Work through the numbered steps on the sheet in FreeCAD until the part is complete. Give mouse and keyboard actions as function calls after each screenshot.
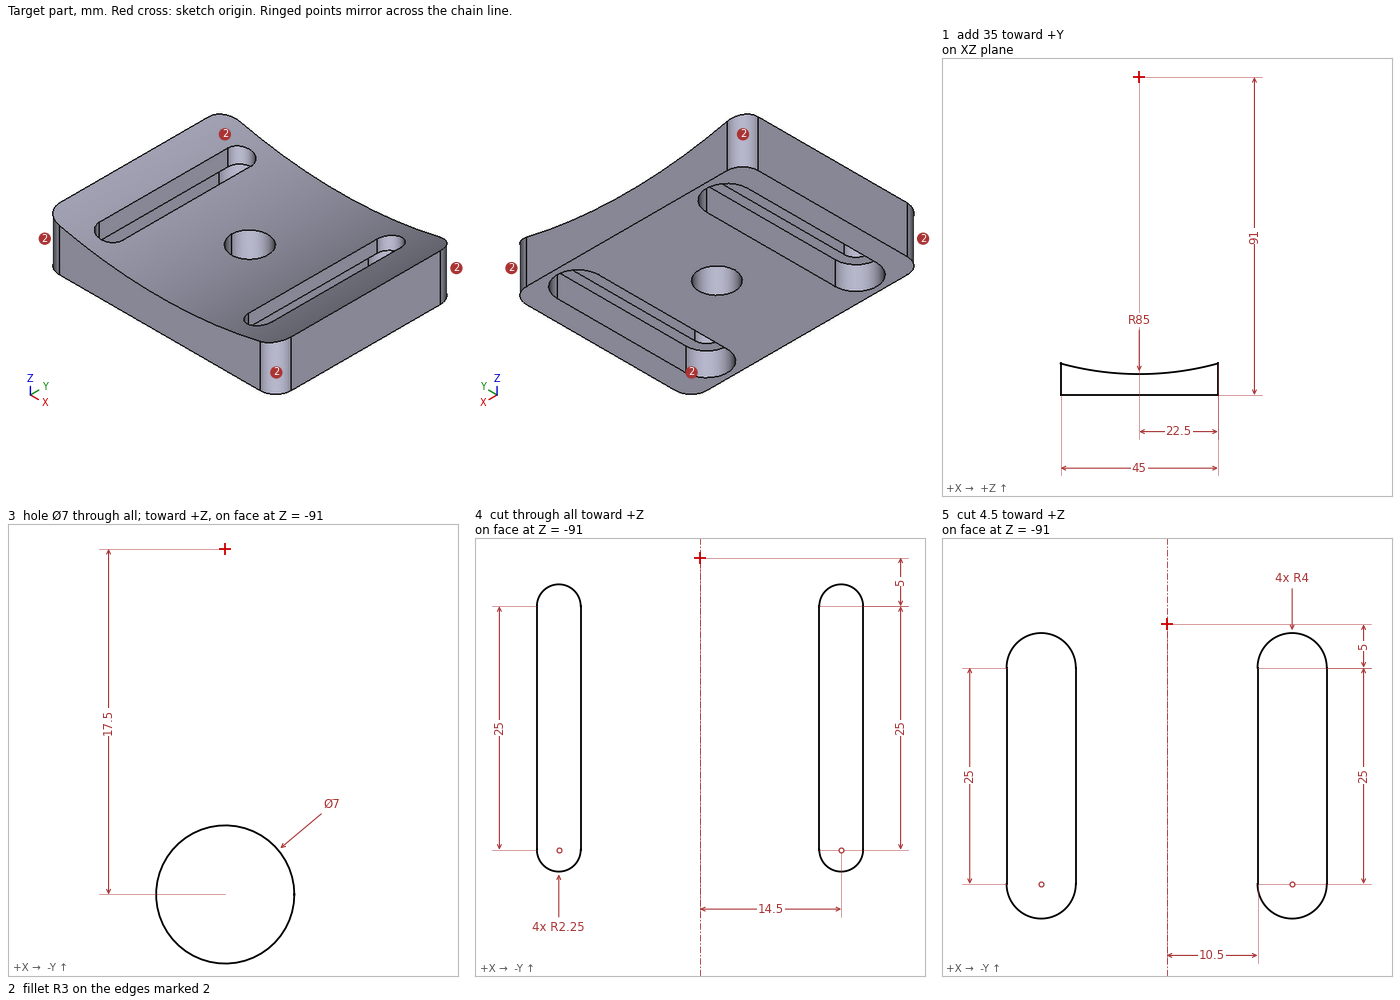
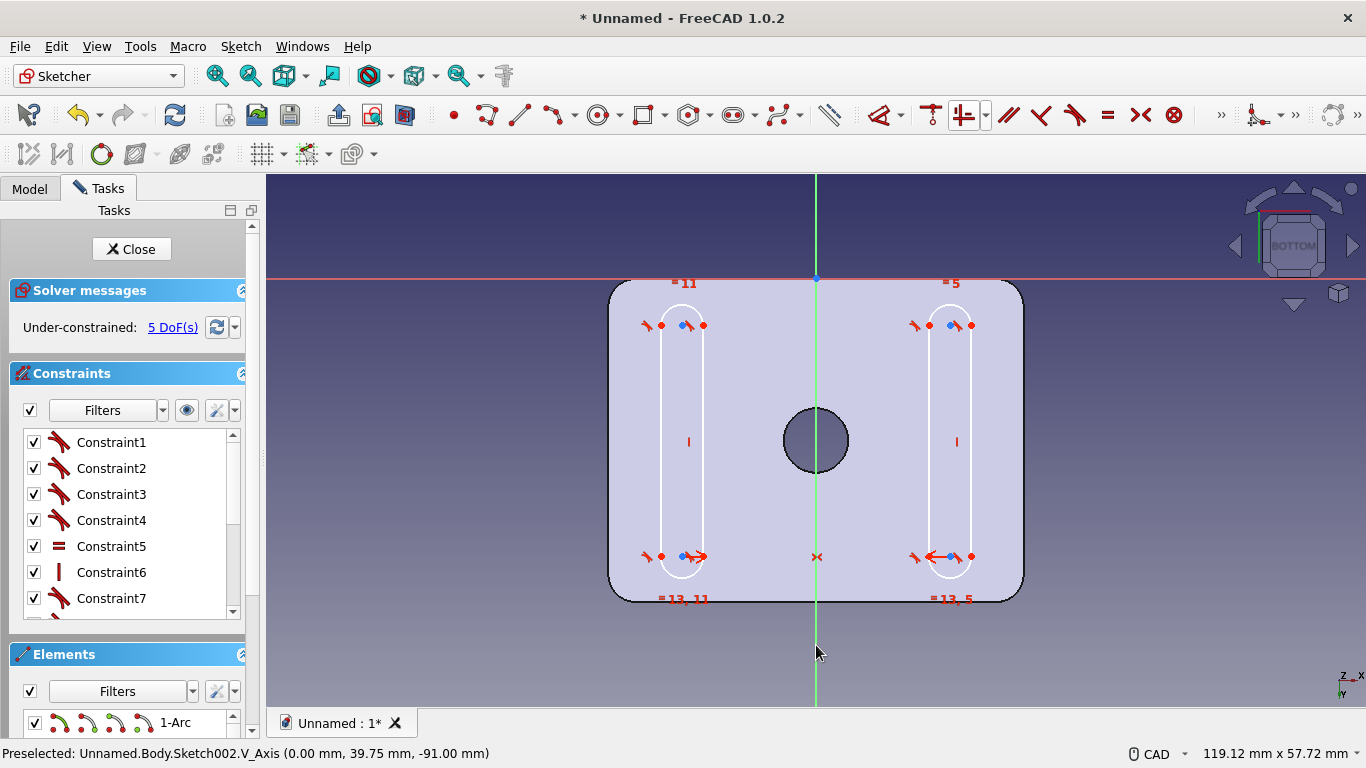
scroll(938, 574, up, 4)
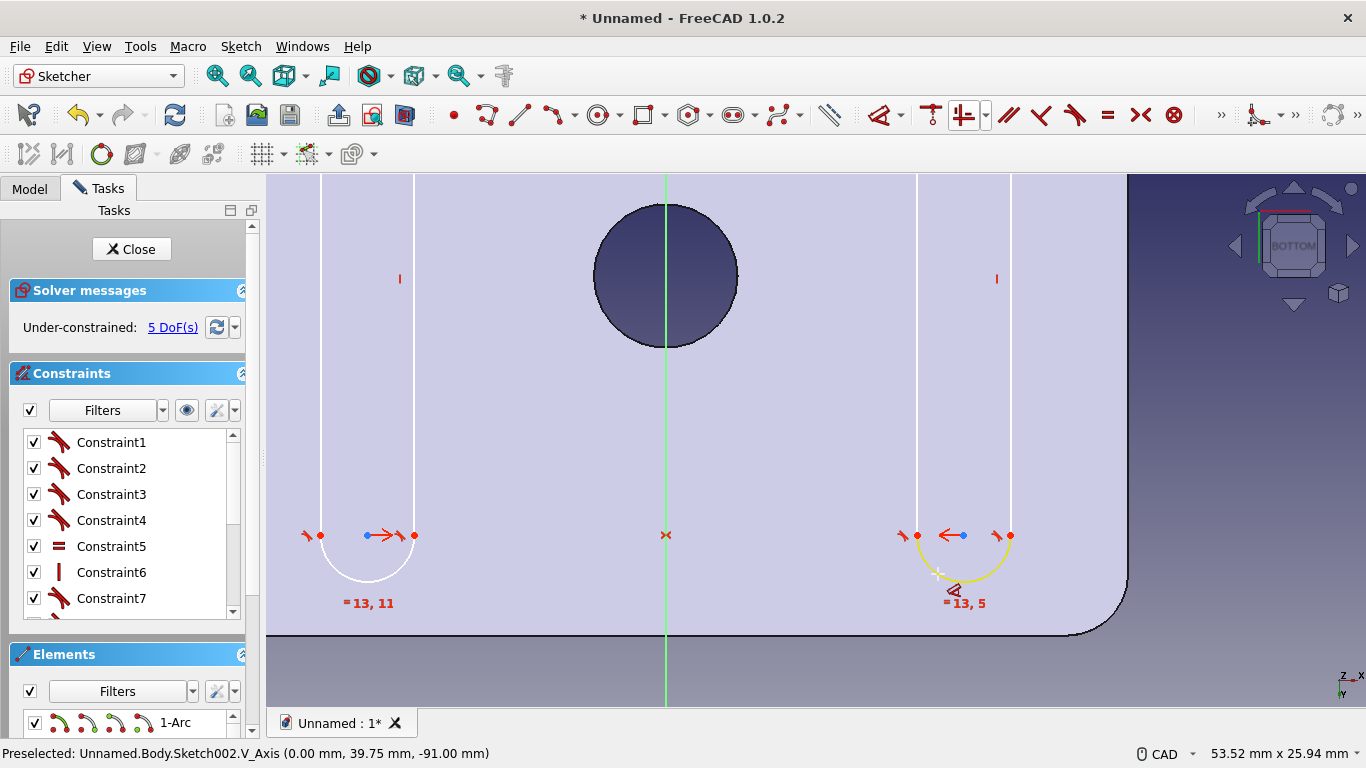
click(936, 573)
click(917, 599)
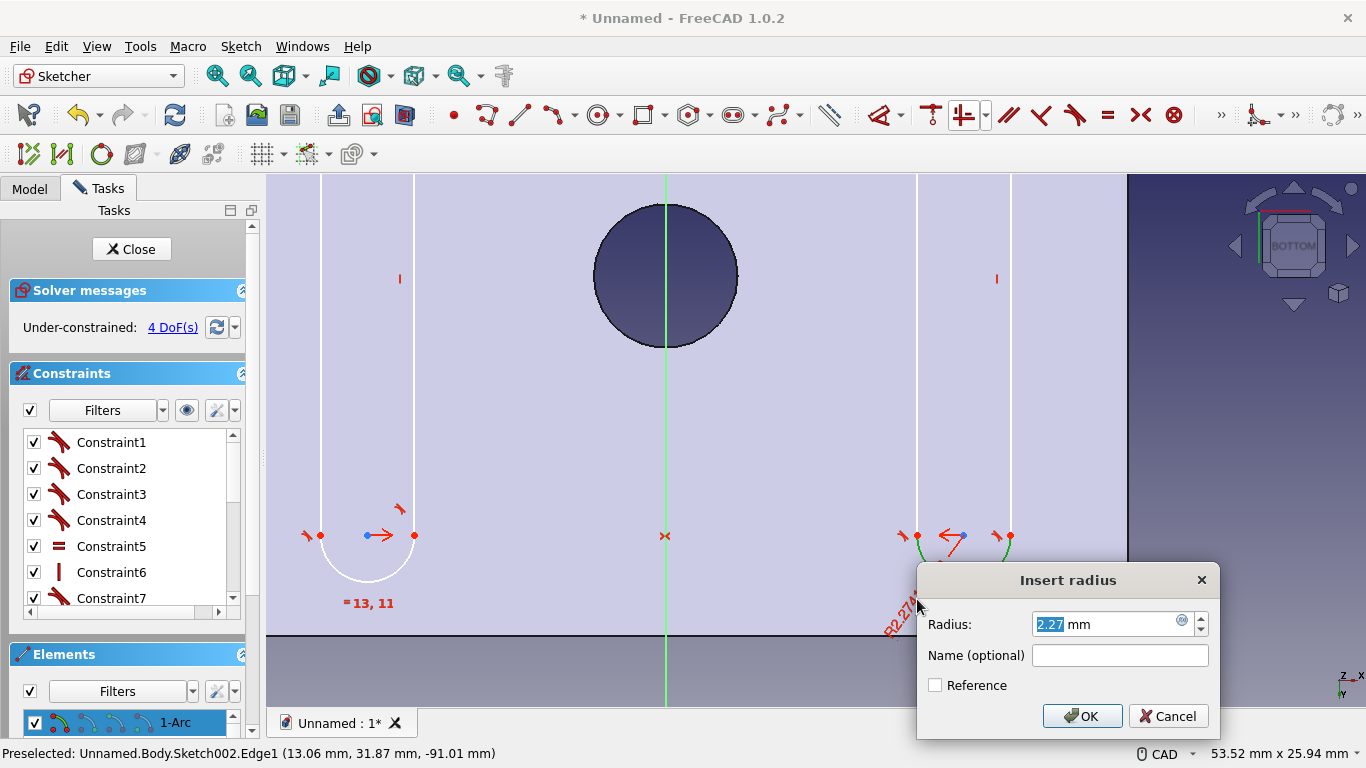
text(2.25)
key(Return)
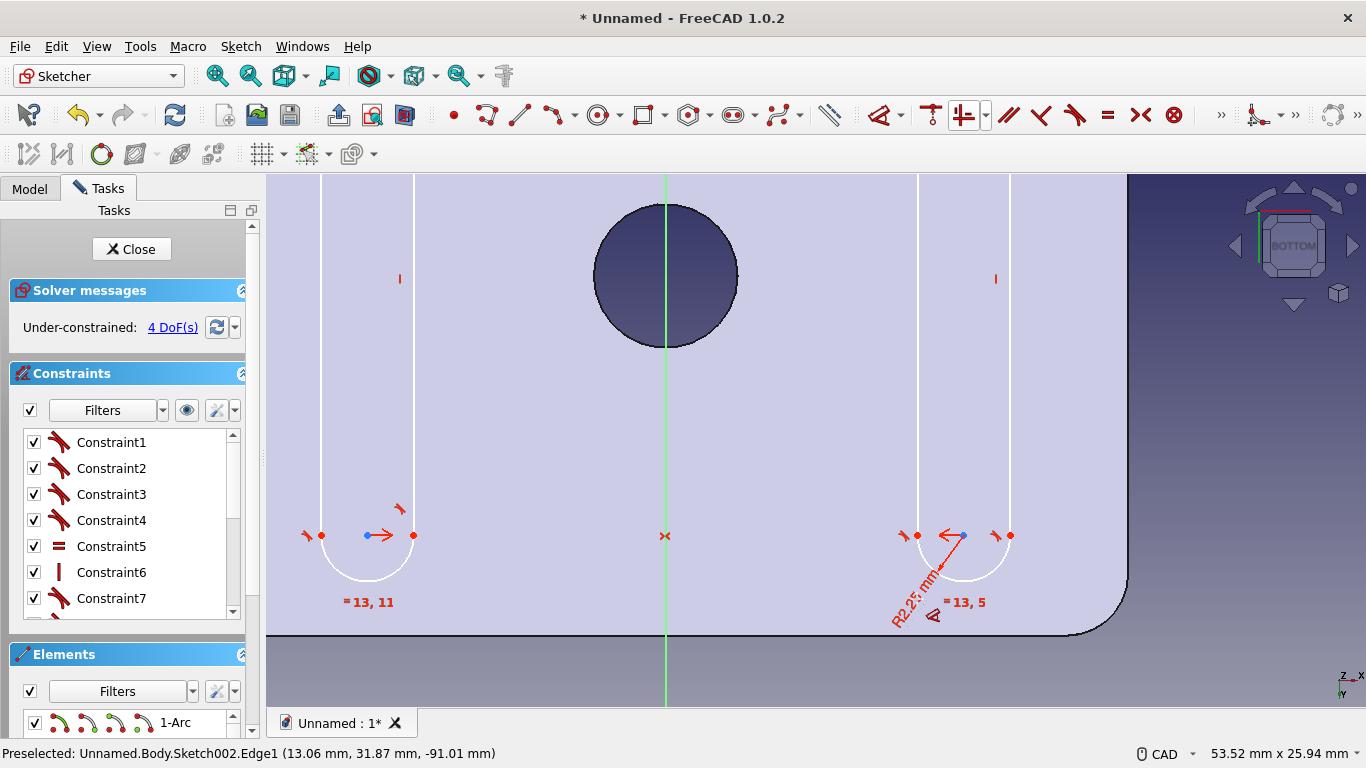
click(918, 381)
click(952, 369)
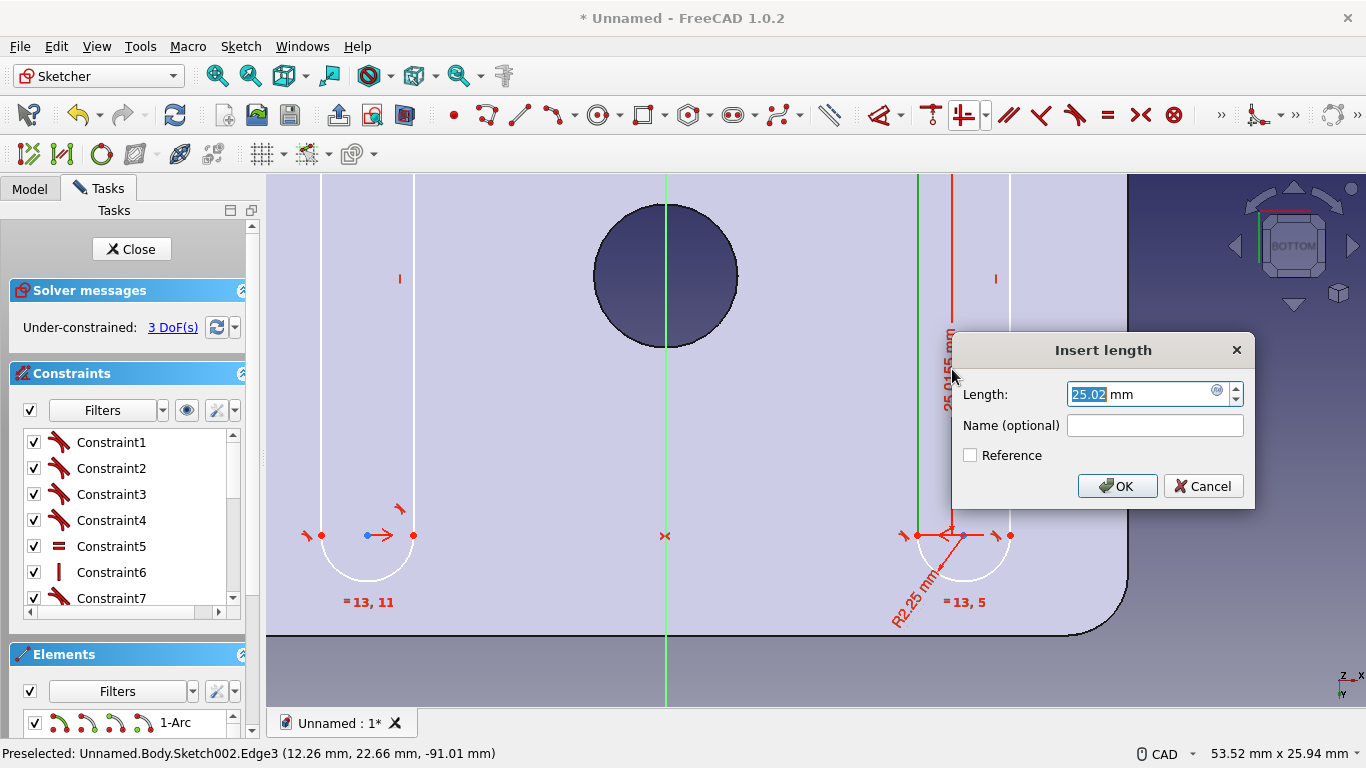
text(25)
key(Return)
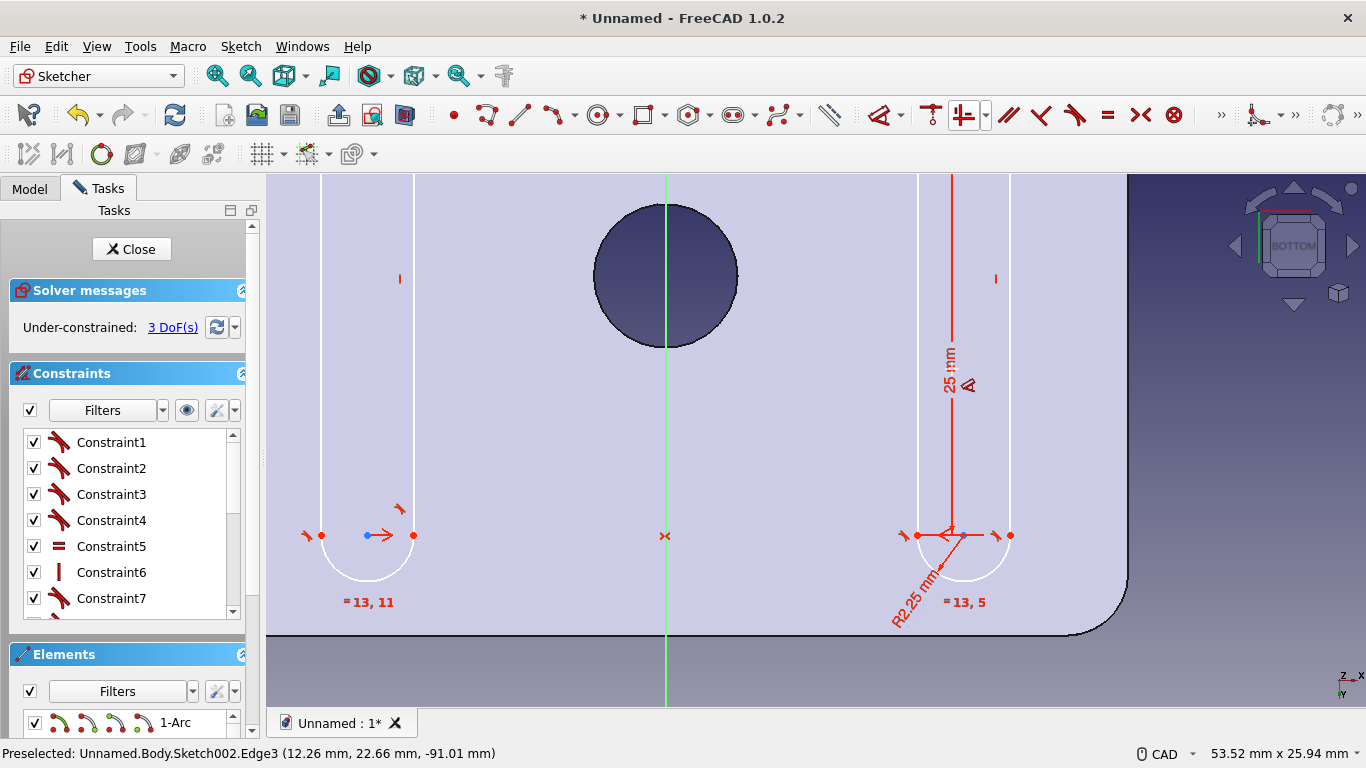
click(321, 381)
click(355, 369)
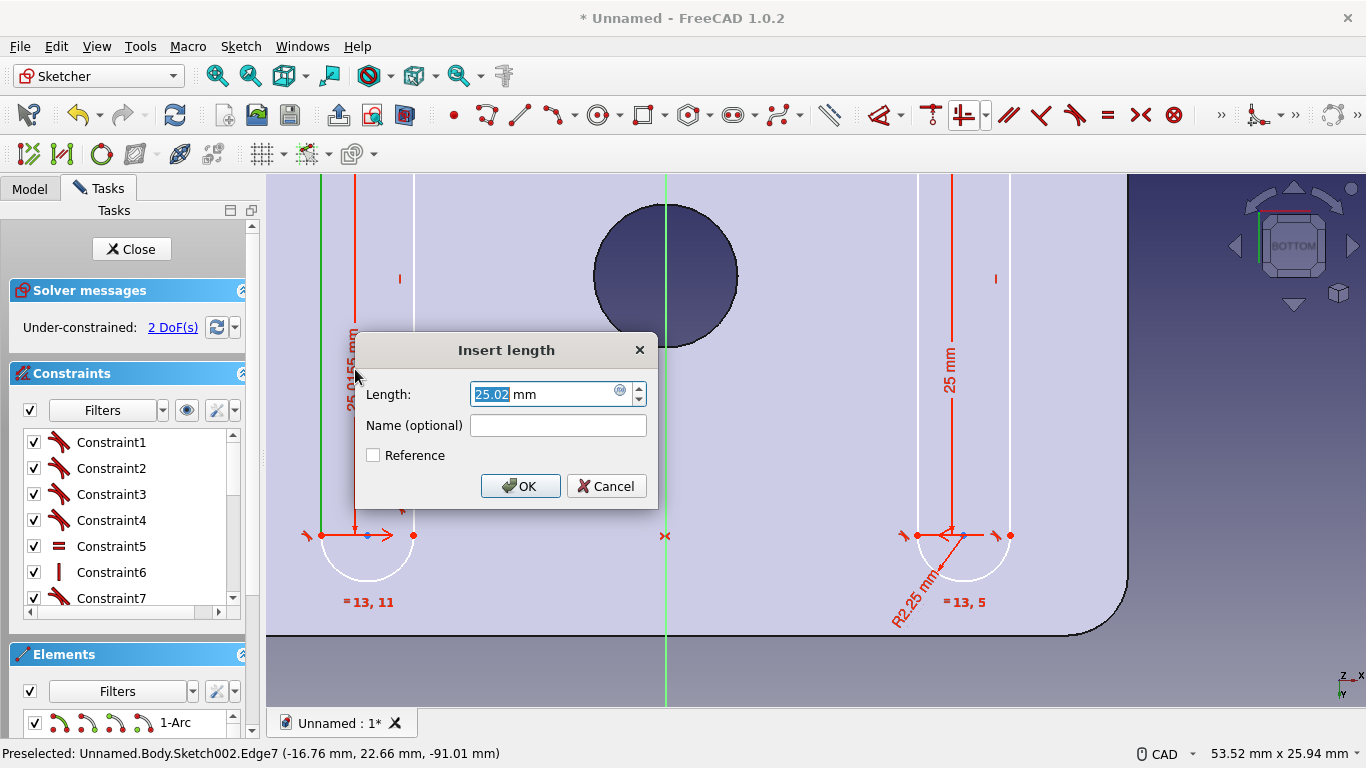
text(25)
key(Return)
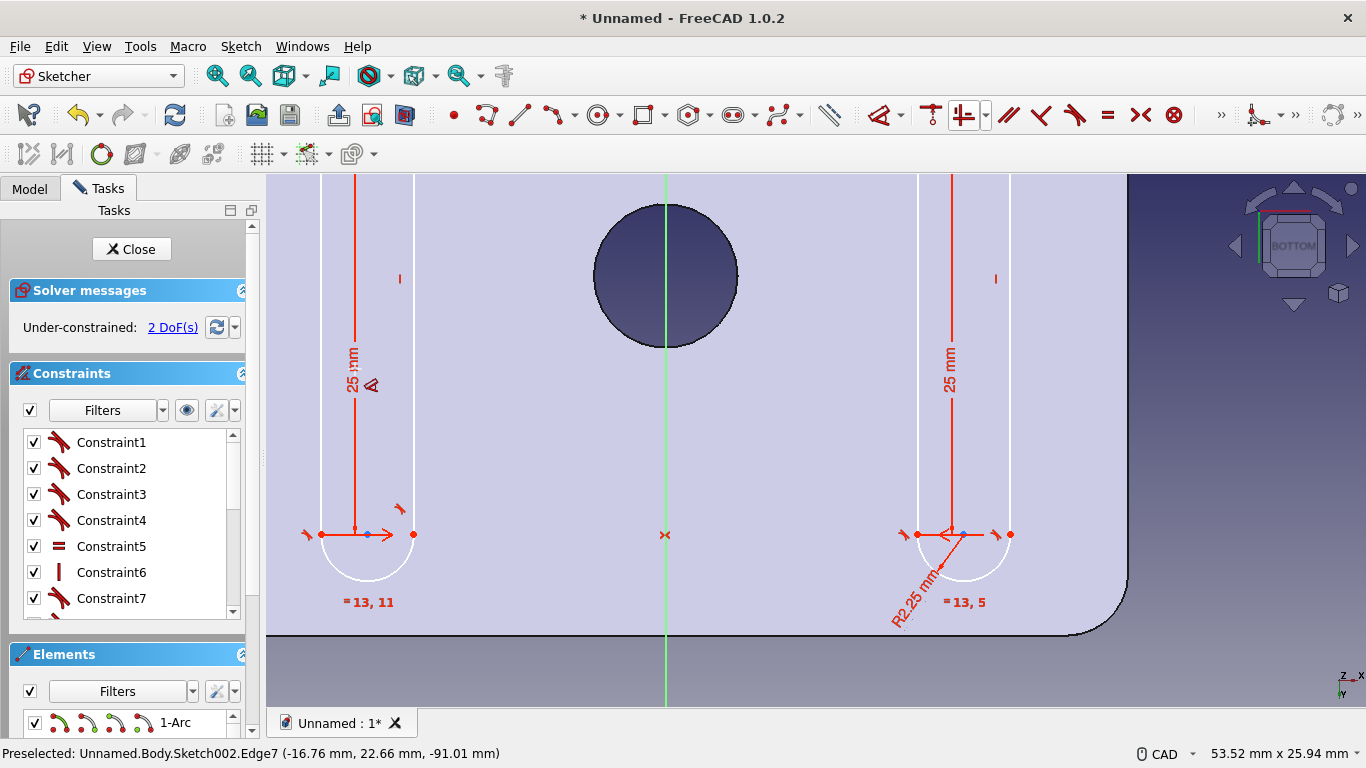
scroll(847, 675, down, 3)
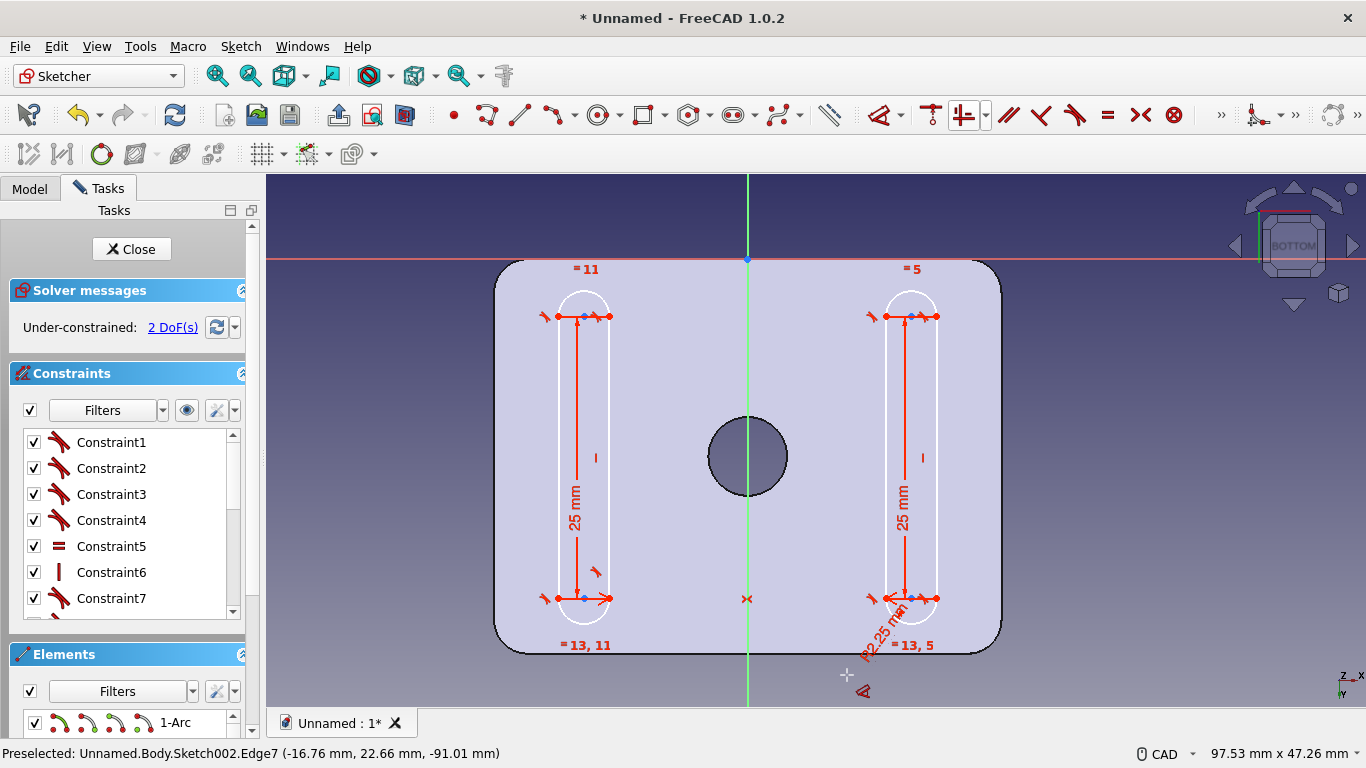
click(937, 317)
click(971, 288)